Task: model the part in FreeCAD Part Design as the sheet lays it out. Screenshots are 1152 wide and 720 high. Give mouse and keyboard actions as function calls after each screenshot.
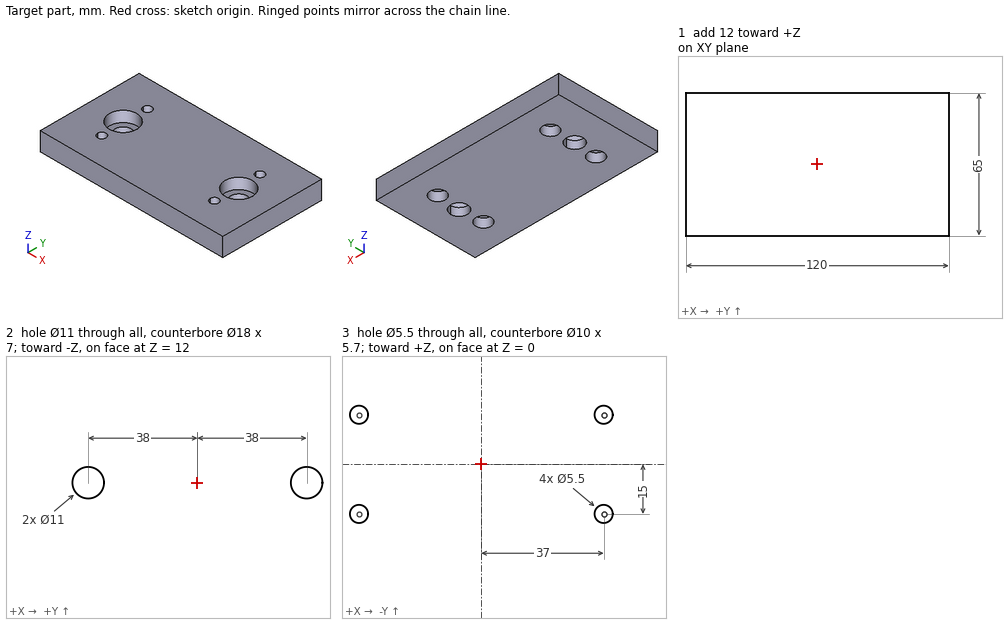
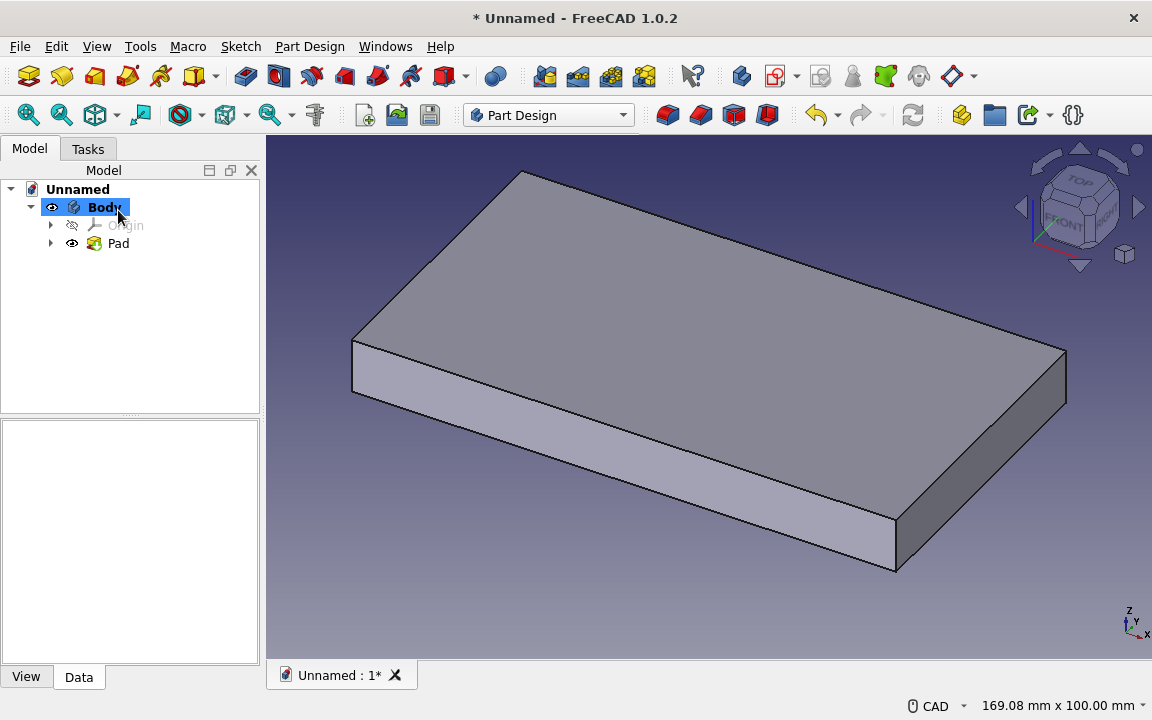
click(787, 370)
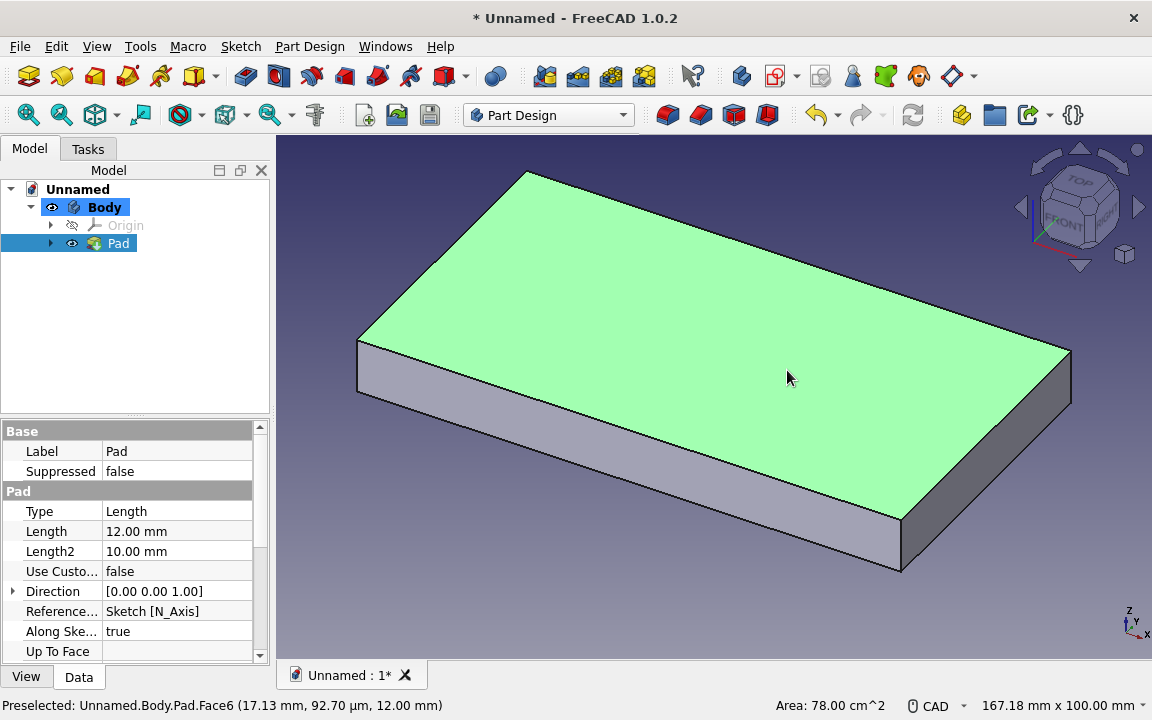
click(774, 76)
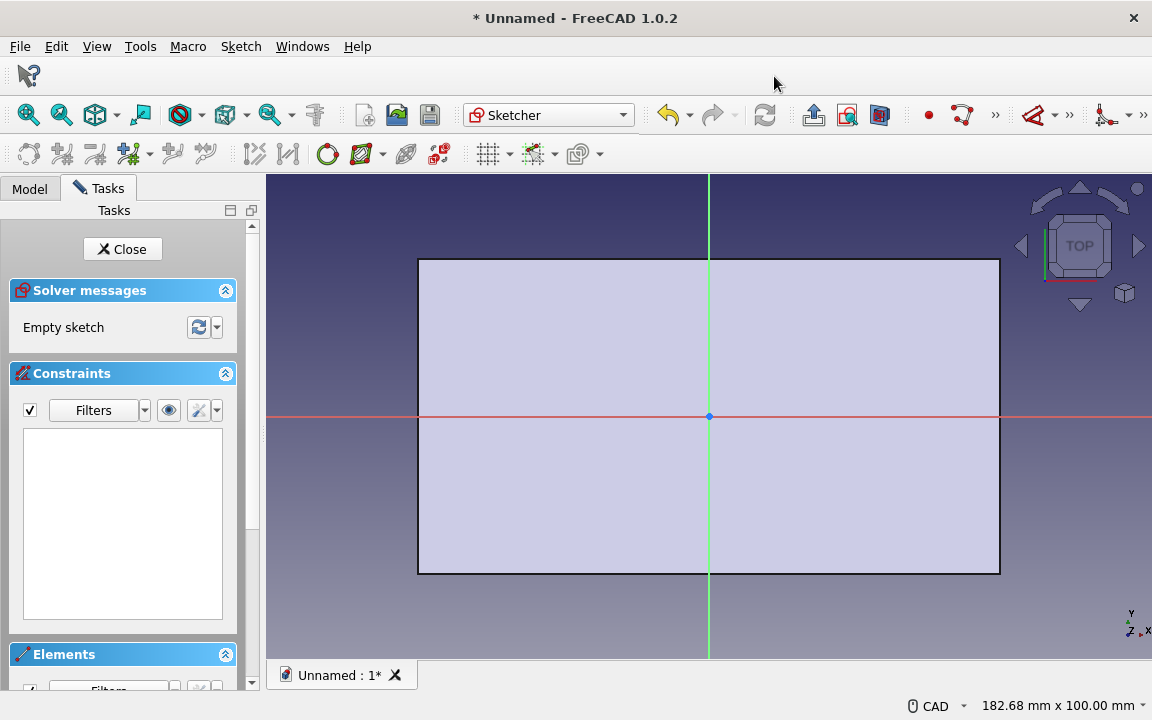
key(g)
key(c)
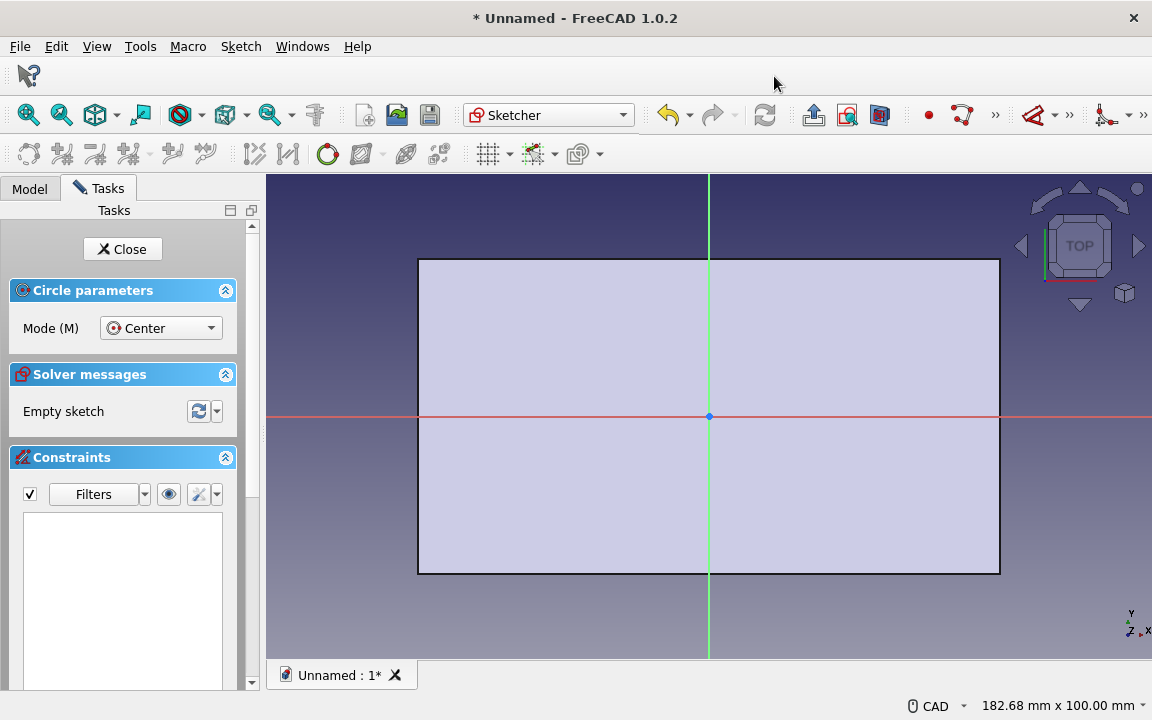
click(525, 416)
move(544, 398)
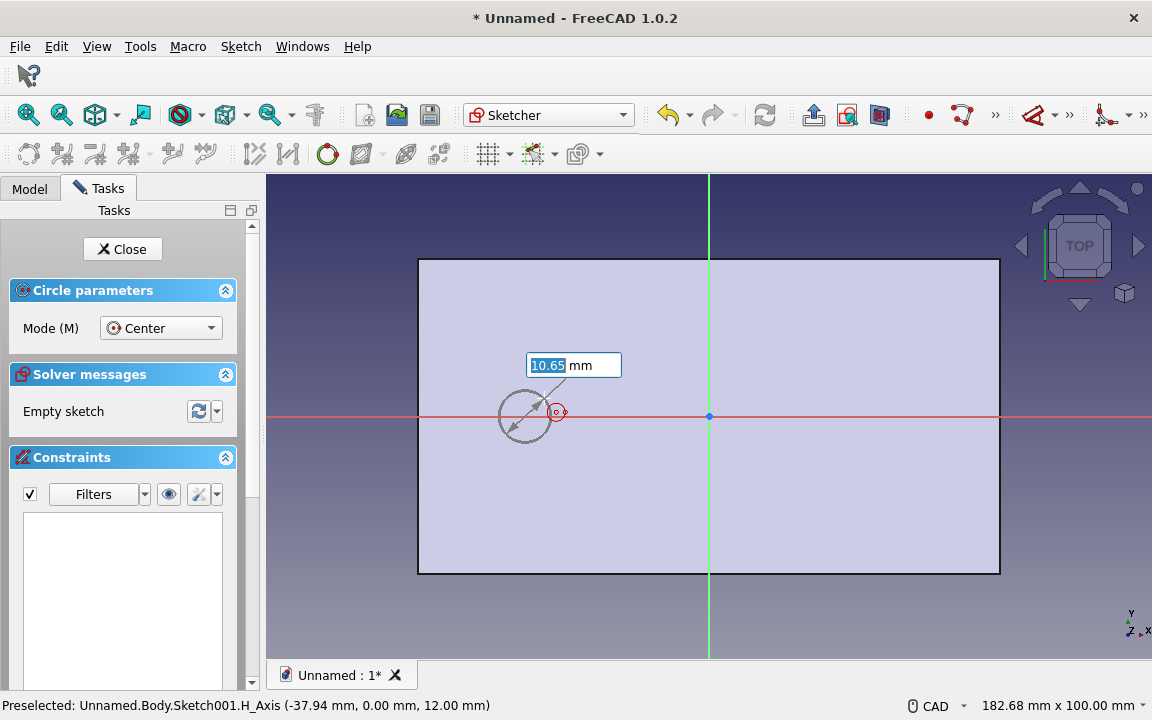
text(11)
key(Return)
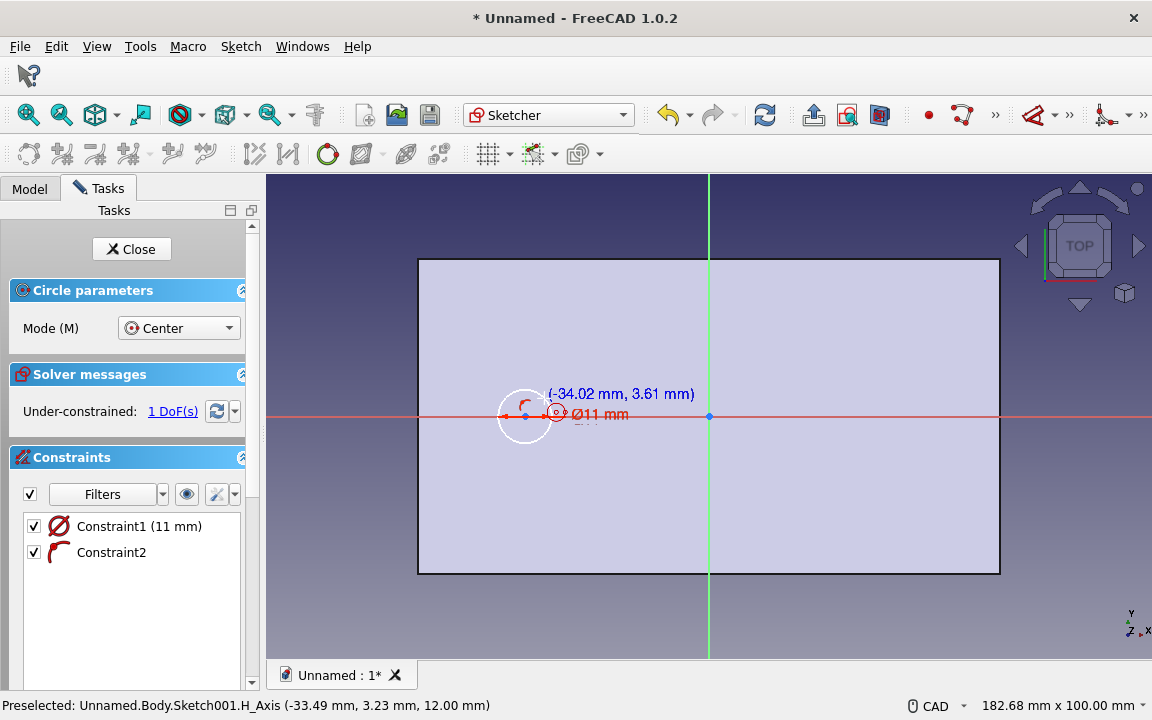
click(893, 416)
move(912, 398)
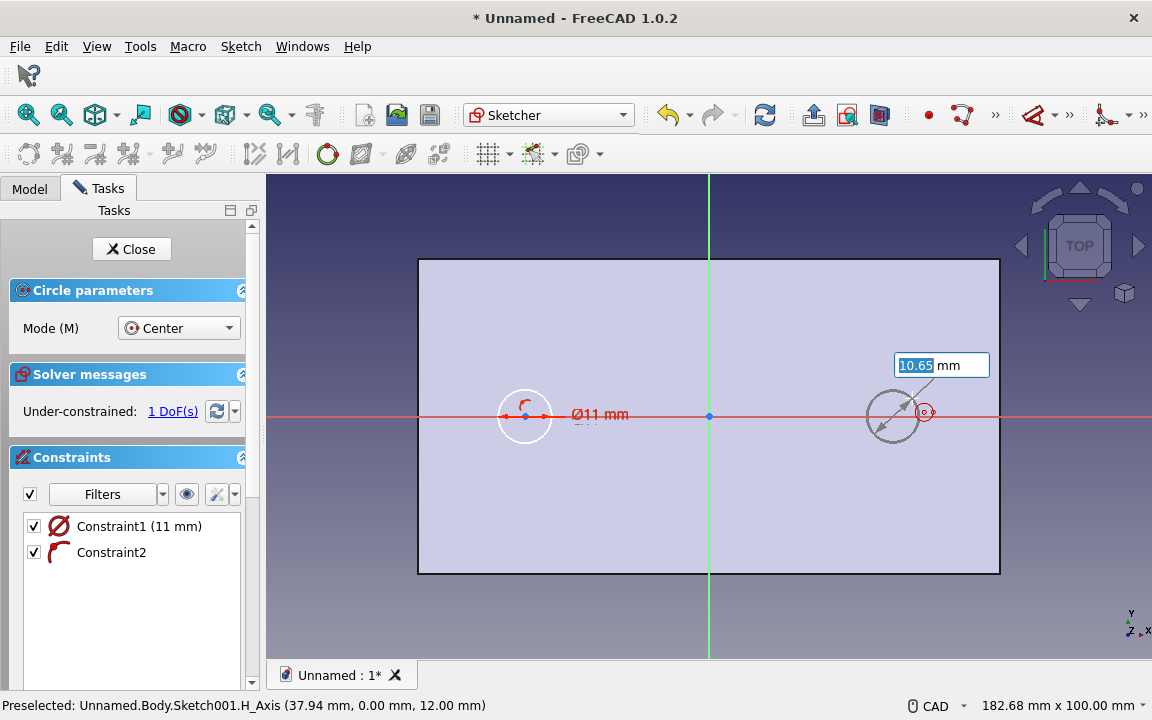
text(11)
key(Return)
key(Escape)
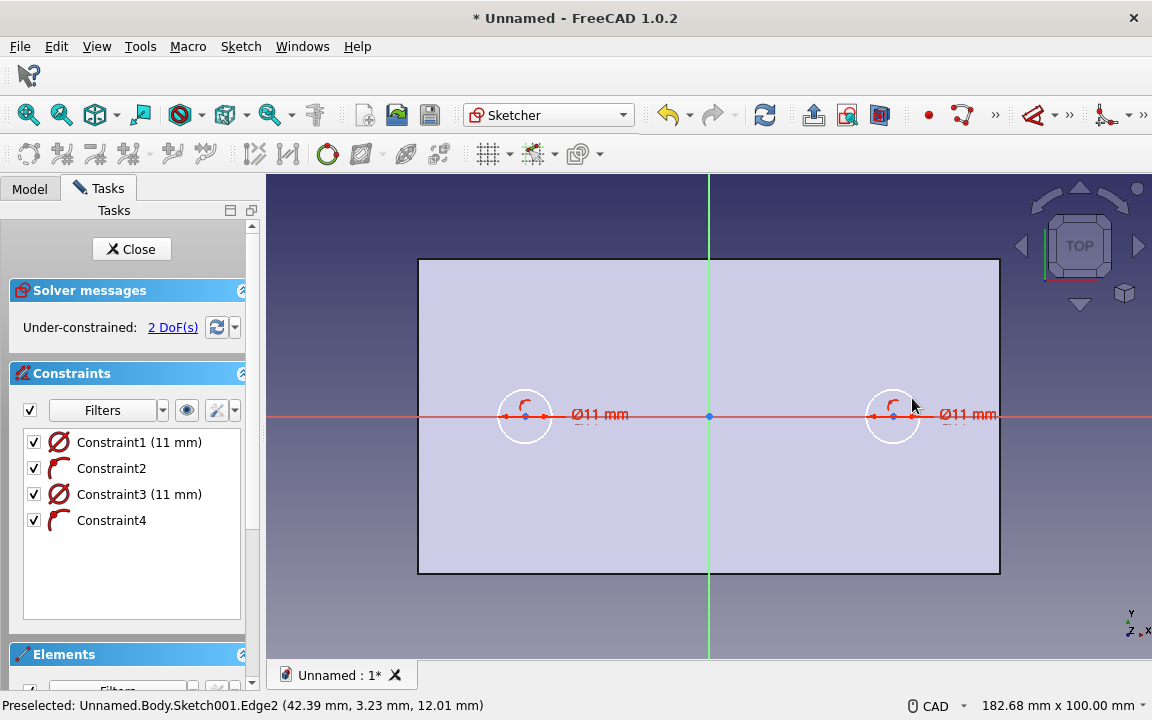
click(1032, 116)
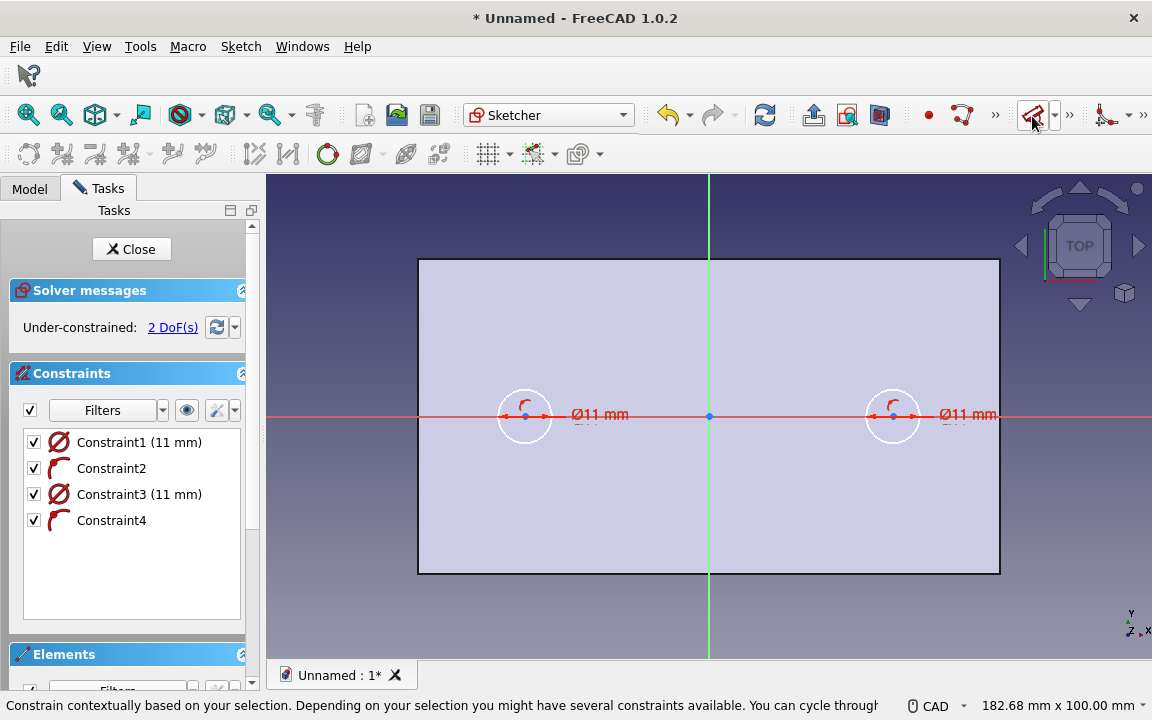
click(525, 416)
click(617, 450)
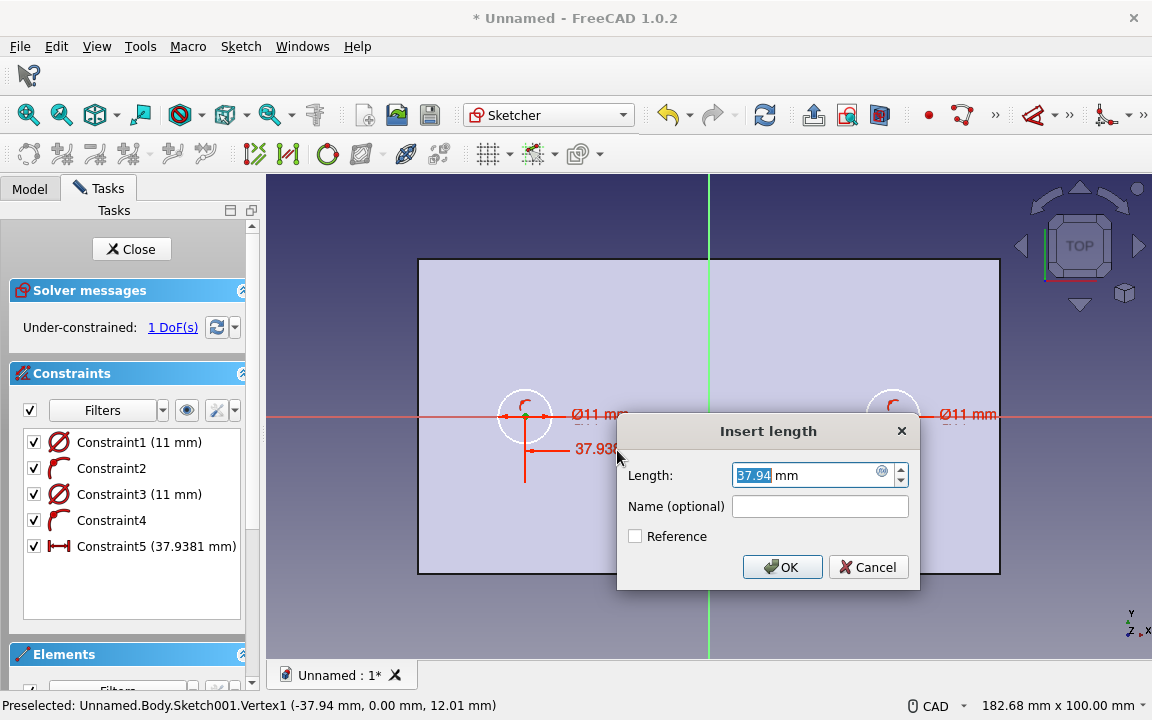
text(38)
key(Return)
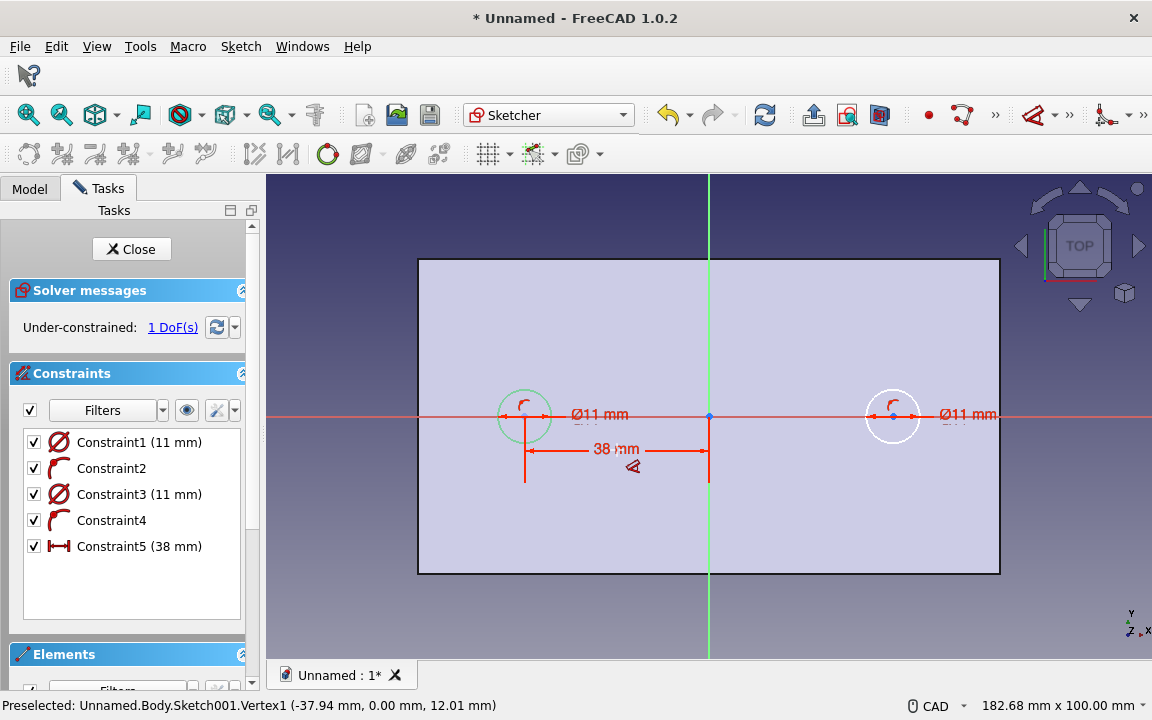
click(893, 416)
click(801, 450)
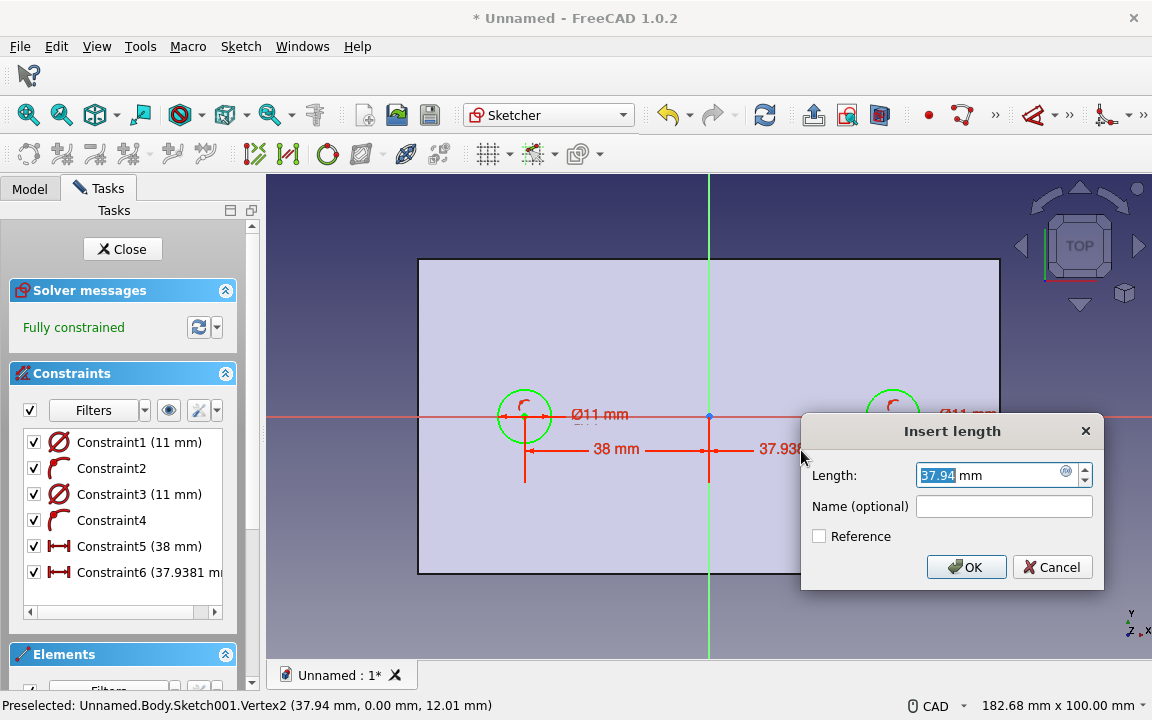
text(38)
key(Return)
key(Escape)